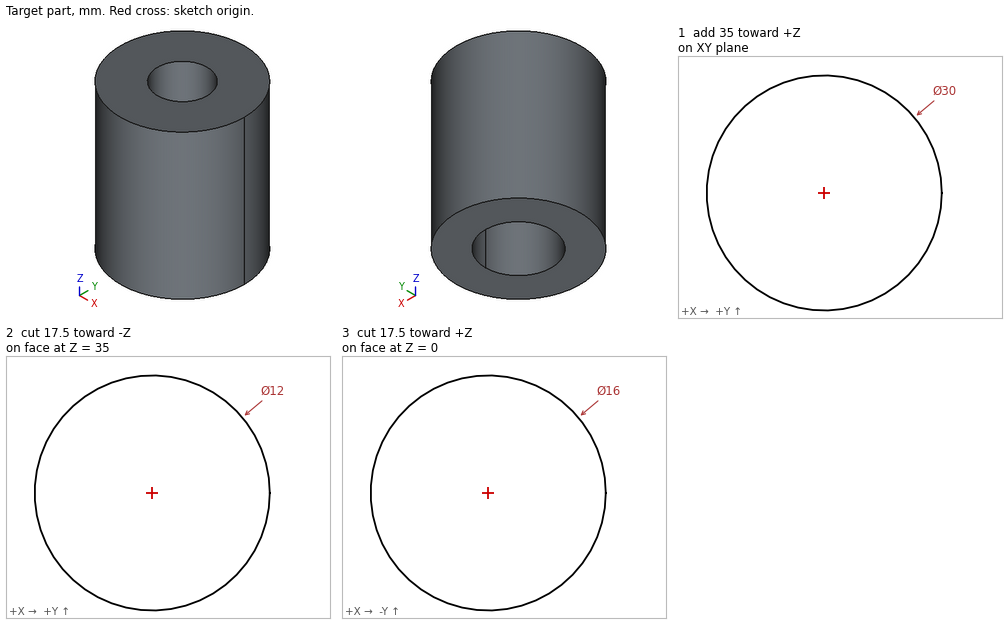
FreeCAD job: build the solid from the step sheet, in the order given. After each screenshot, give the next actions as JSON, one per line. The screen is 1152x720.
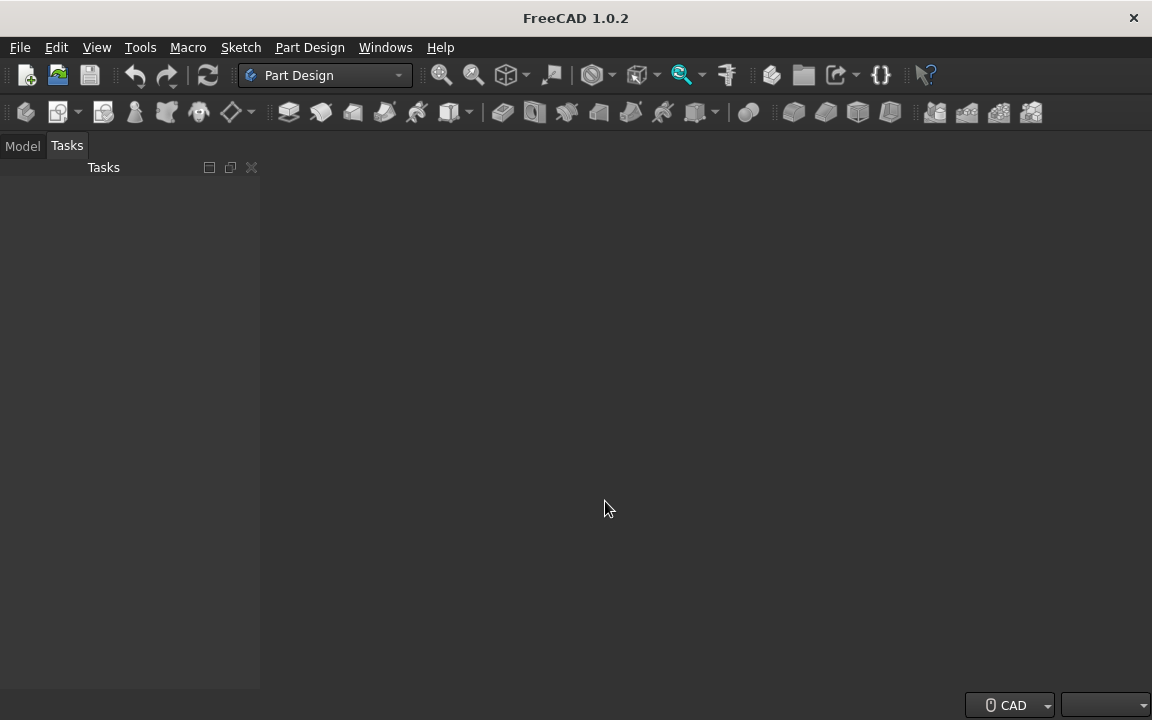
{"action": "key", "text": "ctrl+n"}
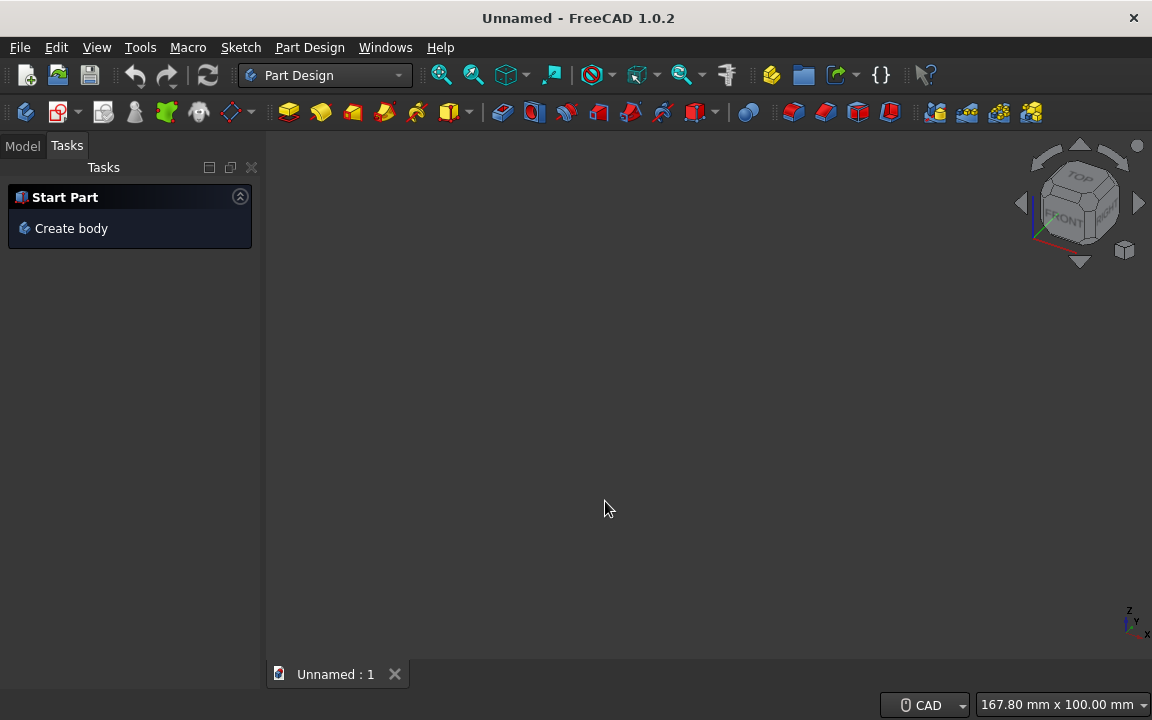
{"action": "left_click", "coordinate": [58, 112]}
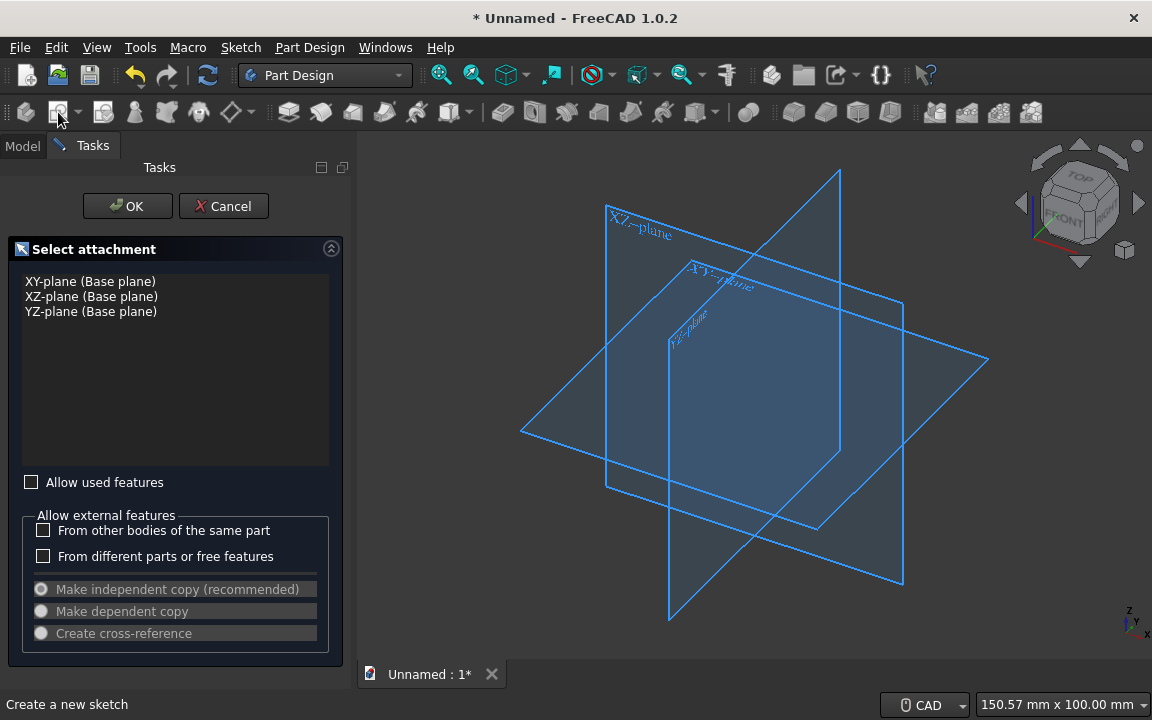
{"action": "left_click", "coordinate": [82, 282]}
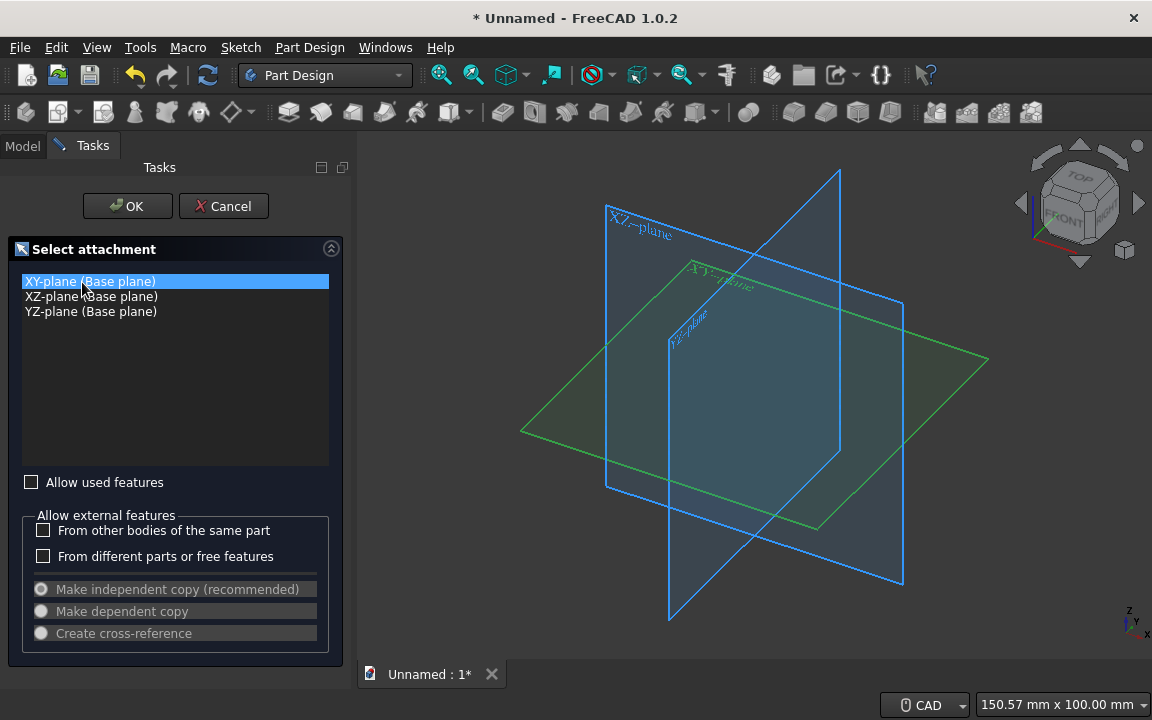
{"action": "left_click", "coordinate": [128, 206]}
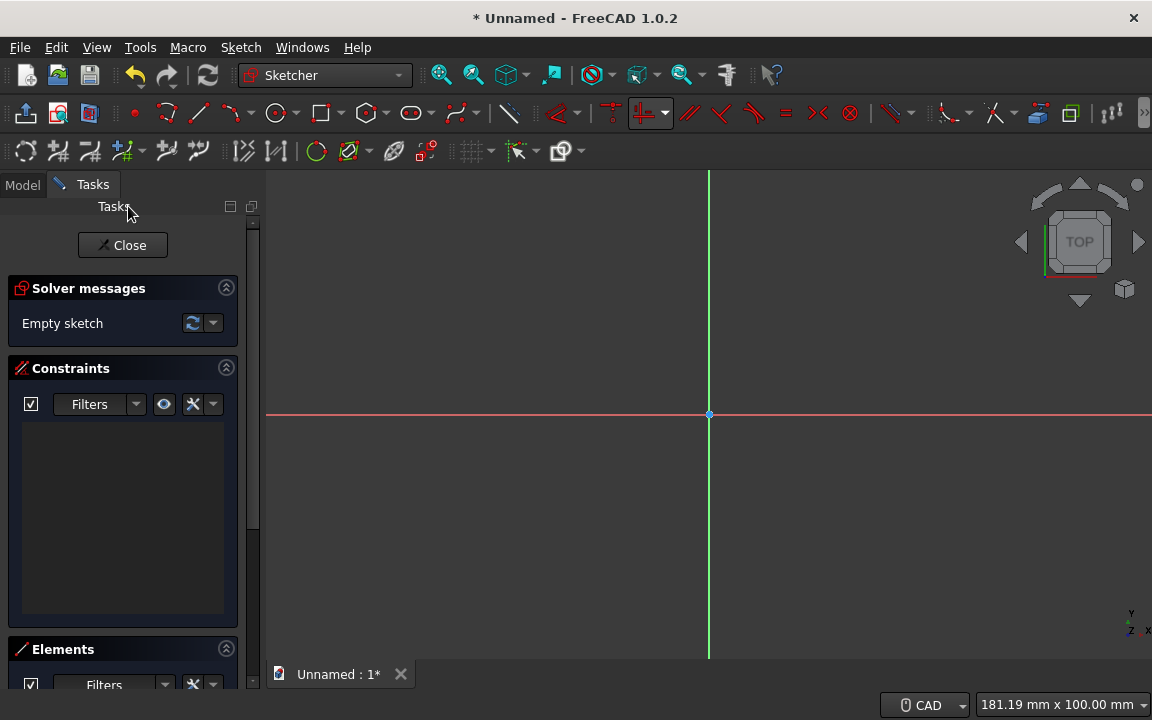
{"action": "scroll", "coordinate": [765, 414], "scroll_direction": "up", "scroll_amount": 4}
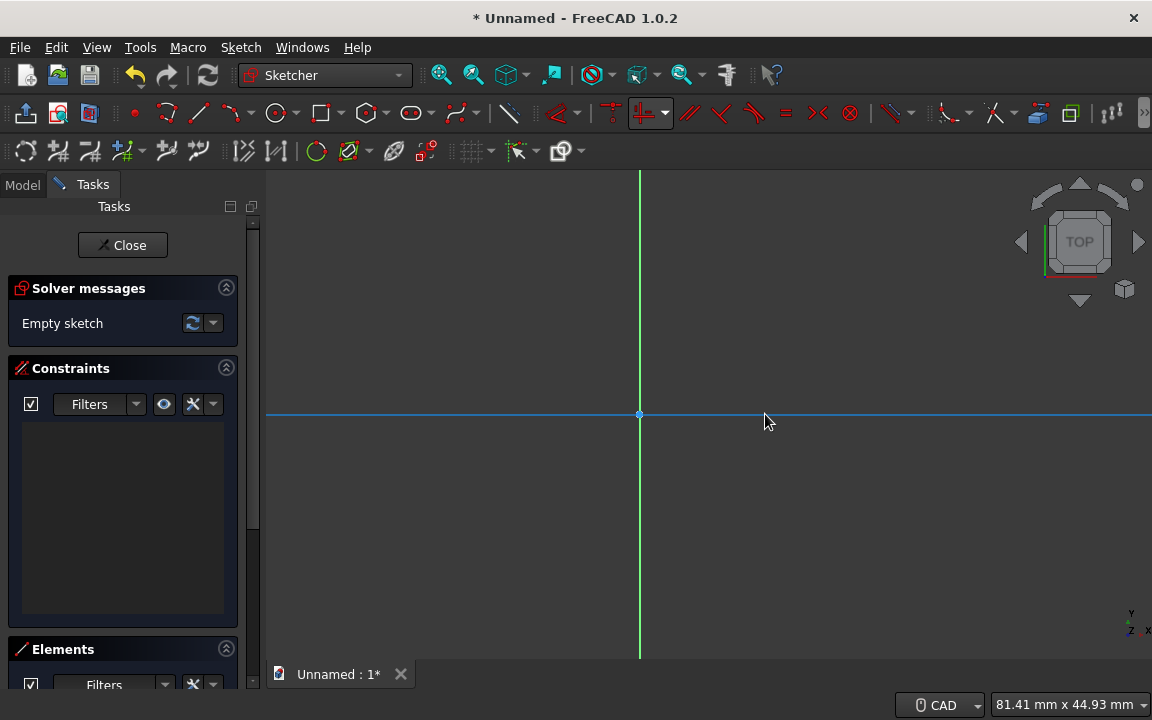
{"action": "key", "text": "g c"}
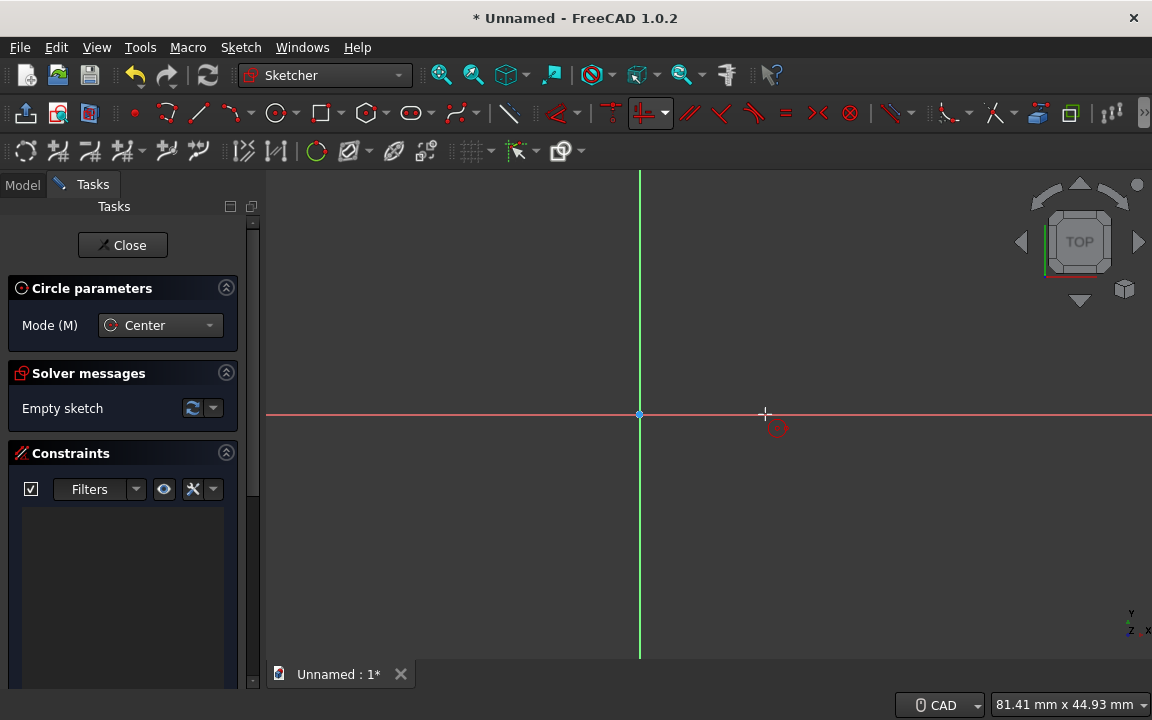
{"action": "left_click", "coordinate": [640, 414]}
{"action": "left_click", "coordinate": [755, 299]}
{"action": "key", "text": "Escape"}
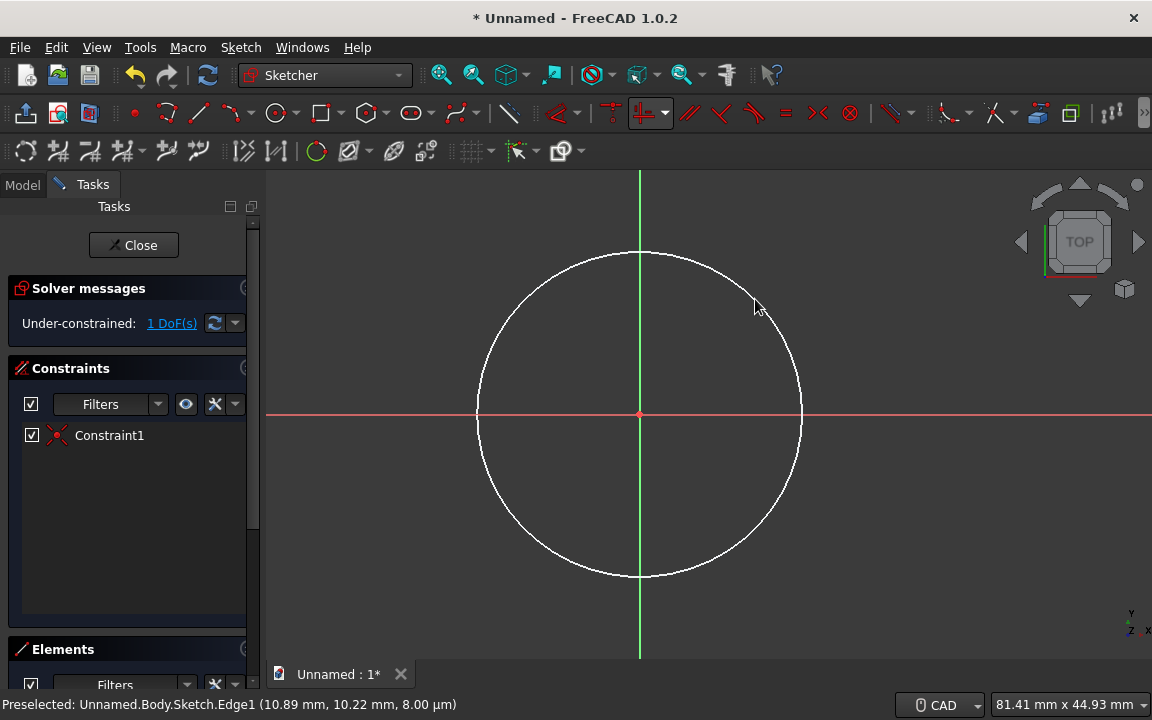
{"action": "key", "text": "d"}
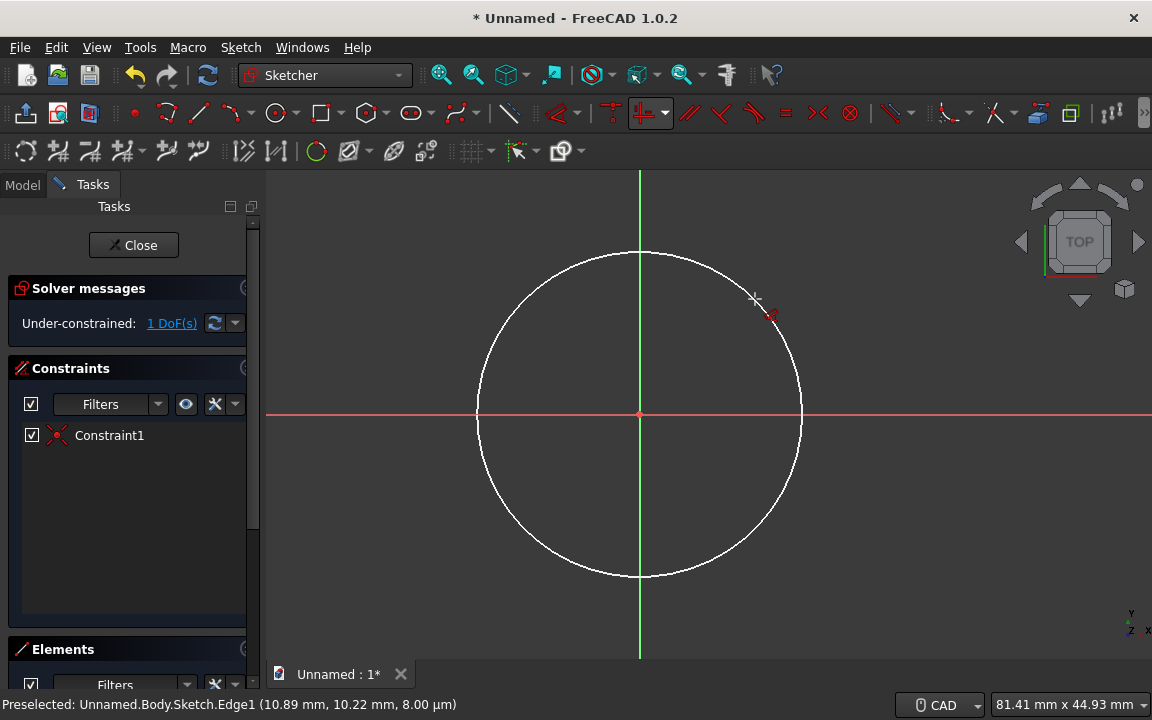
{"action": "left_click", "coordinate": [754, 299]}
{"action": "left_click", "coordinate": [777, 276]}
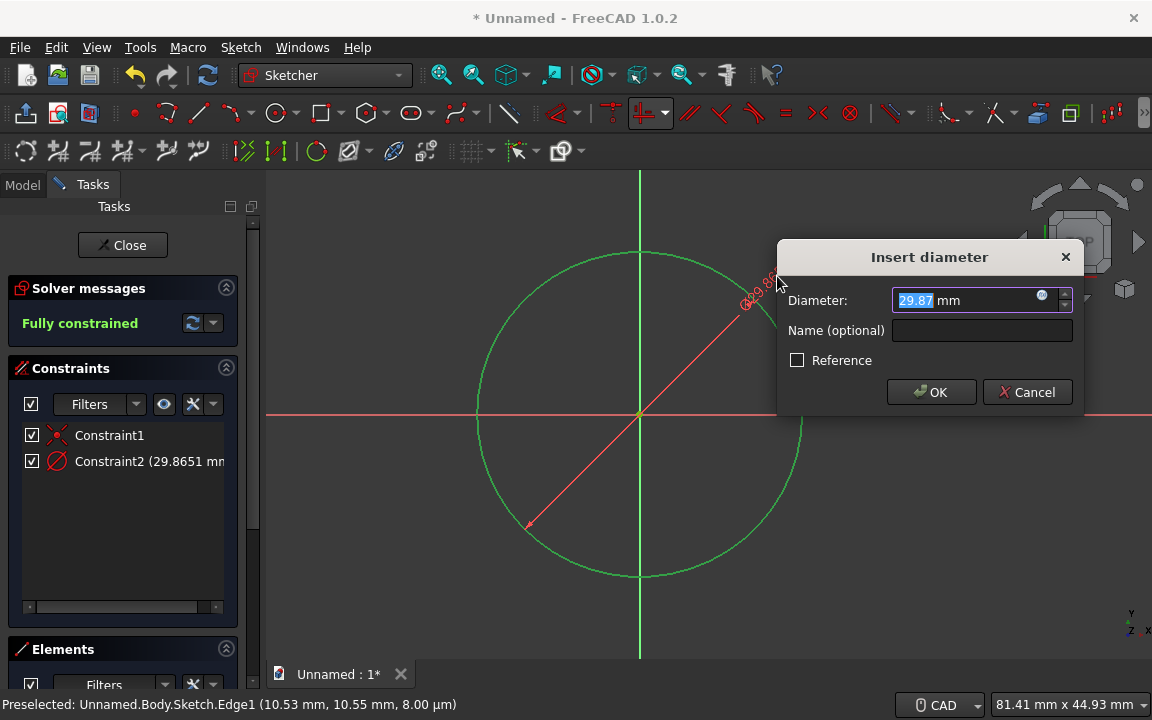
{"action": "type", "text": "30"}
{"action": "key", "text": "Return"}
{"action": "key", "text": "Escape"}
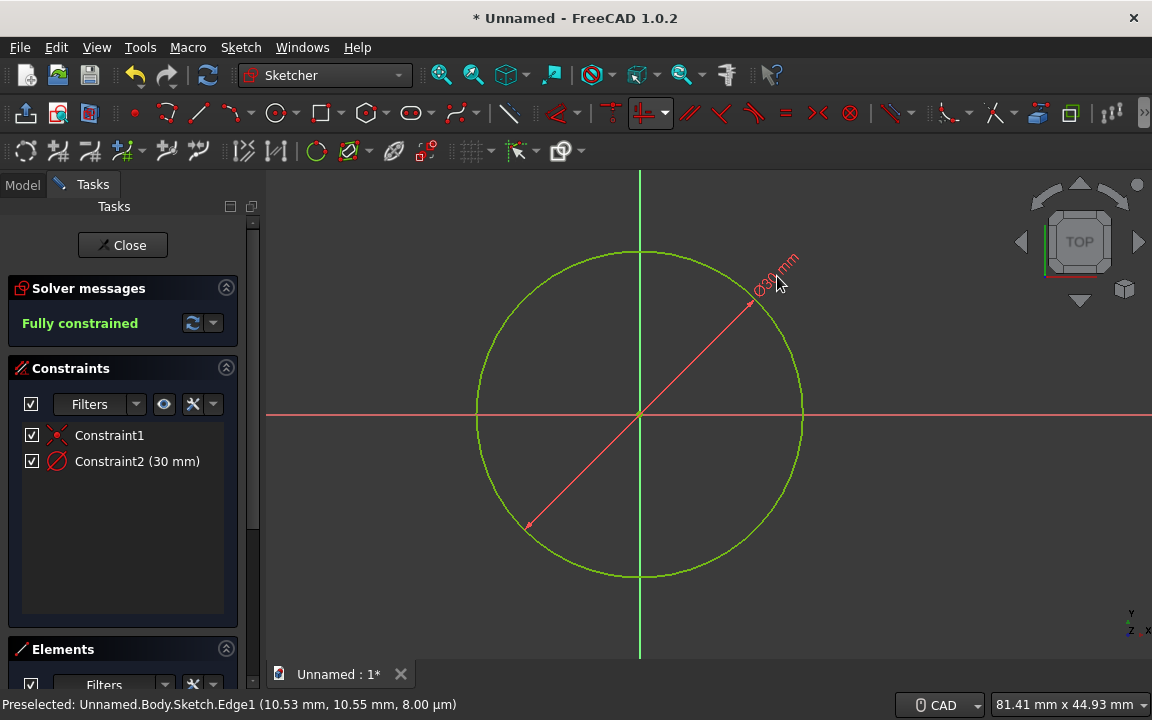
{"action": "left_click", "coordinate": [123, 245]}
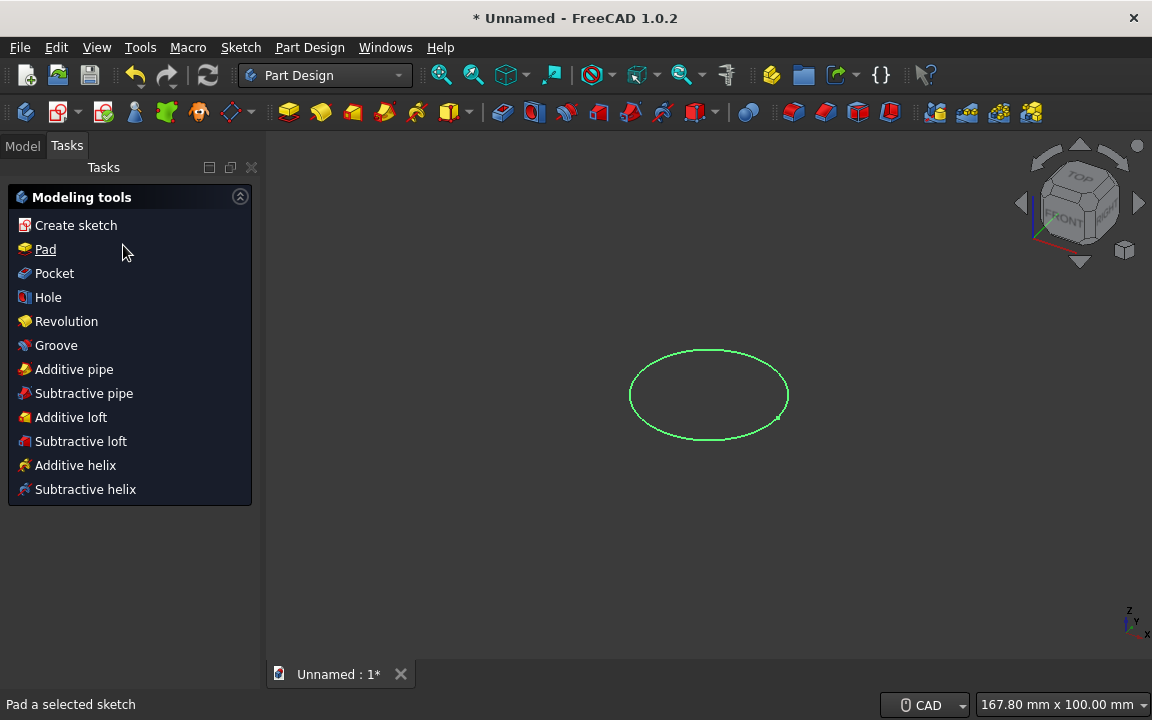
{"action": "left_click", "coordinate": [290, 112]}